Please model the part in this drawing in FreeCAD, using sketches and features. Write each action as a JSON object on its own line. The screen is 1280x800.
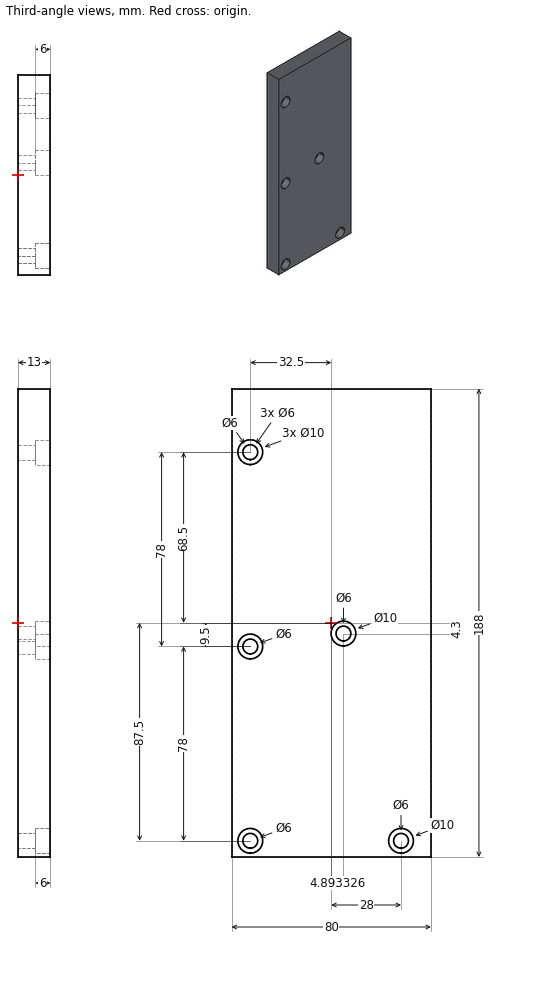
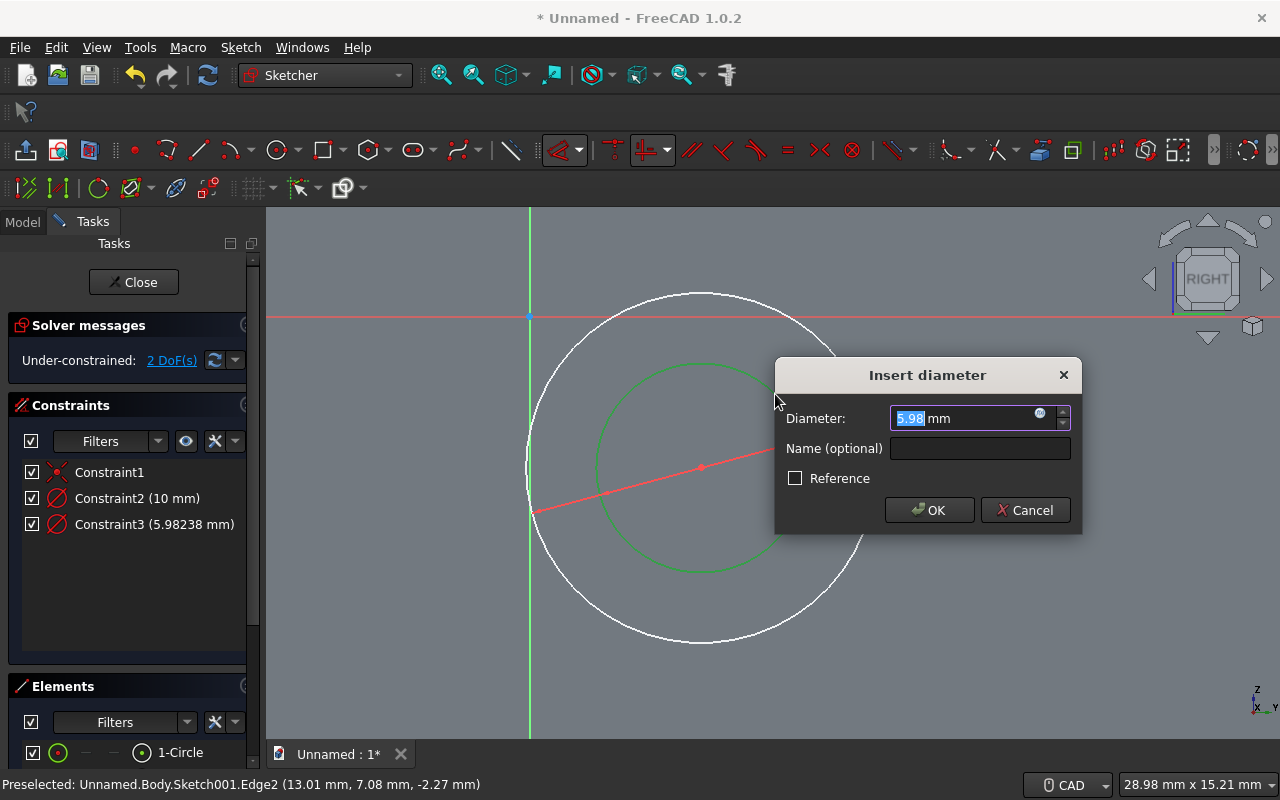
{"action": "type", "text": "6"}
{"action": "key", "text": "Return"}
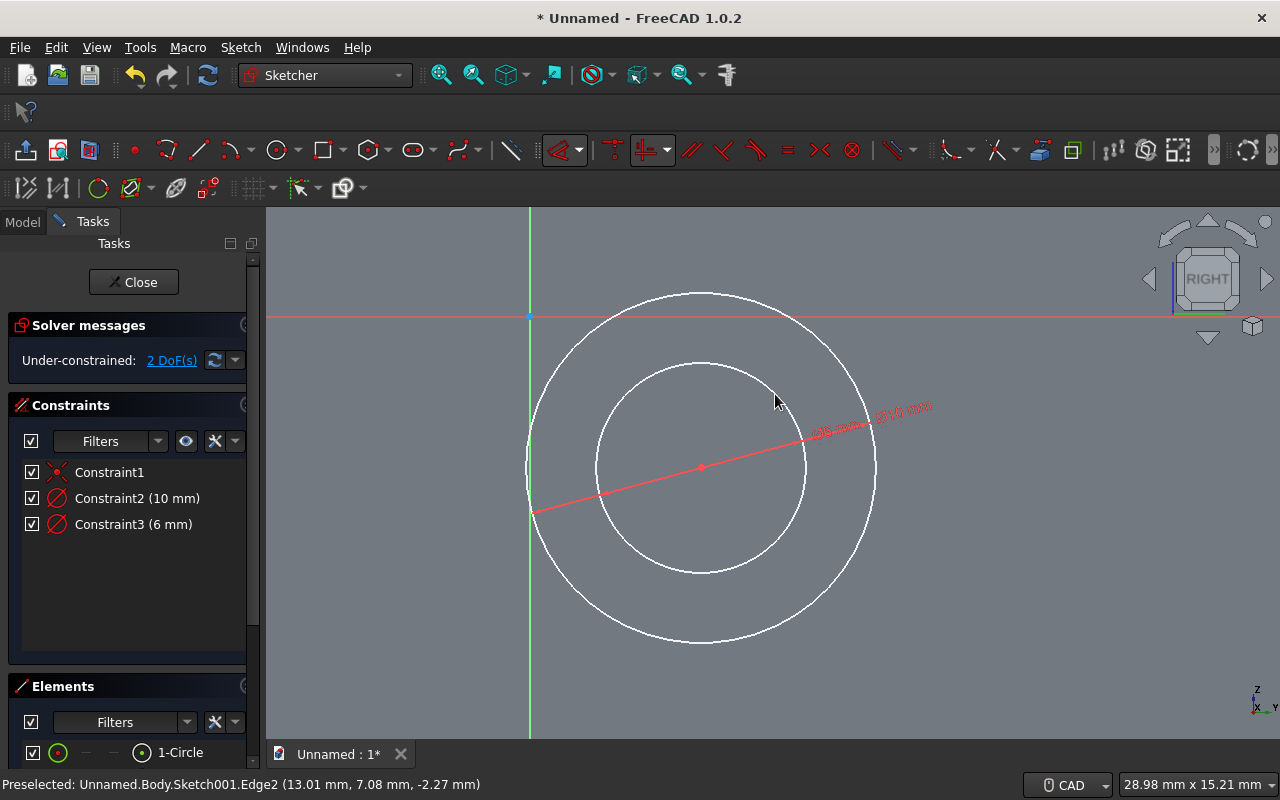
{"action": "left_click", "coordinate": [701, 468]}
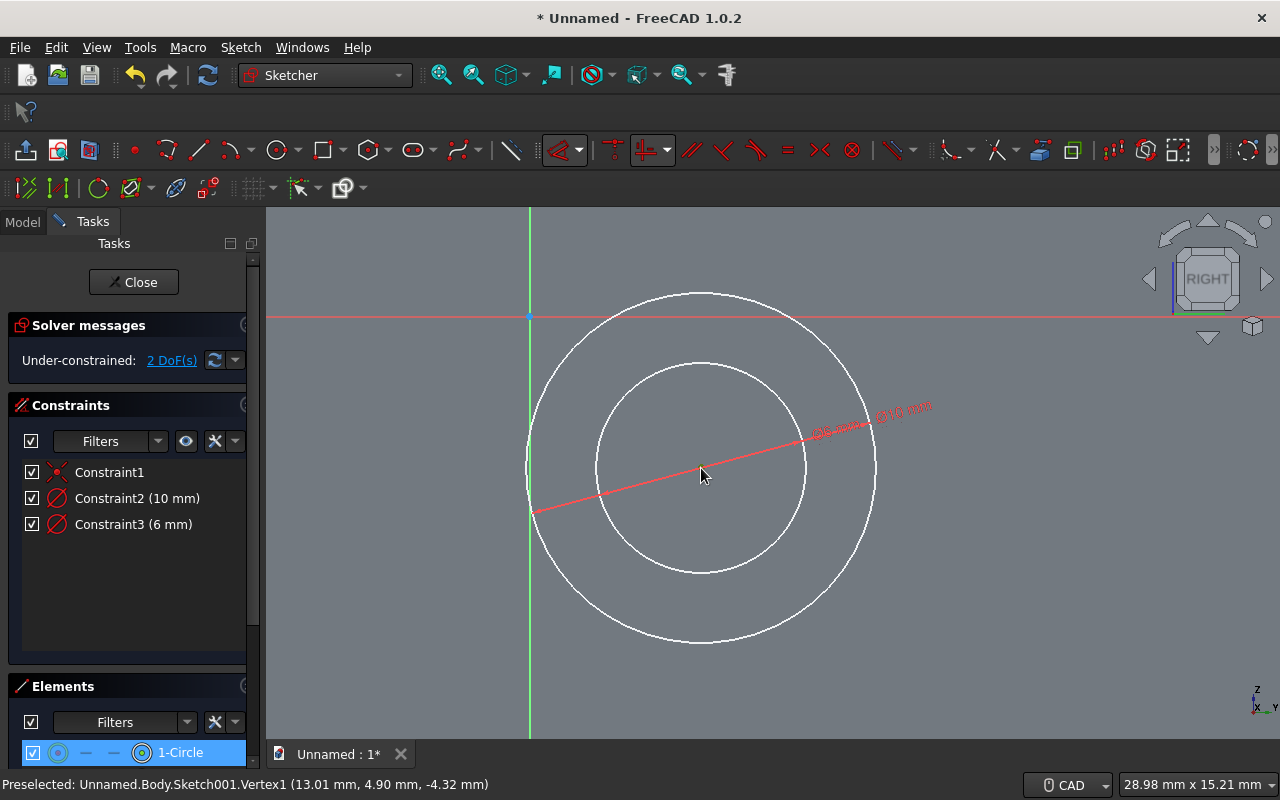
{"action": "key", "text": "i"}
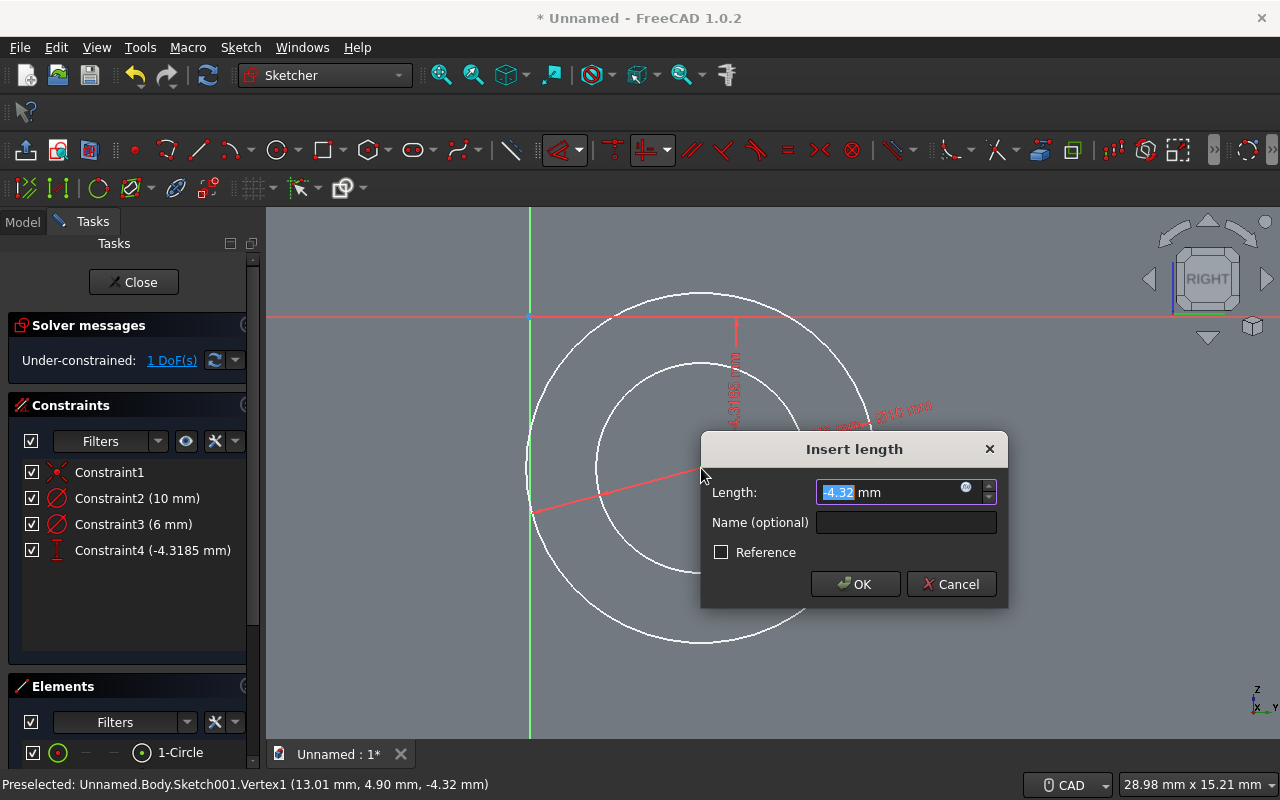
{"action": "type", "text": "-4.3"}
{"action": "key", "text": "Return"}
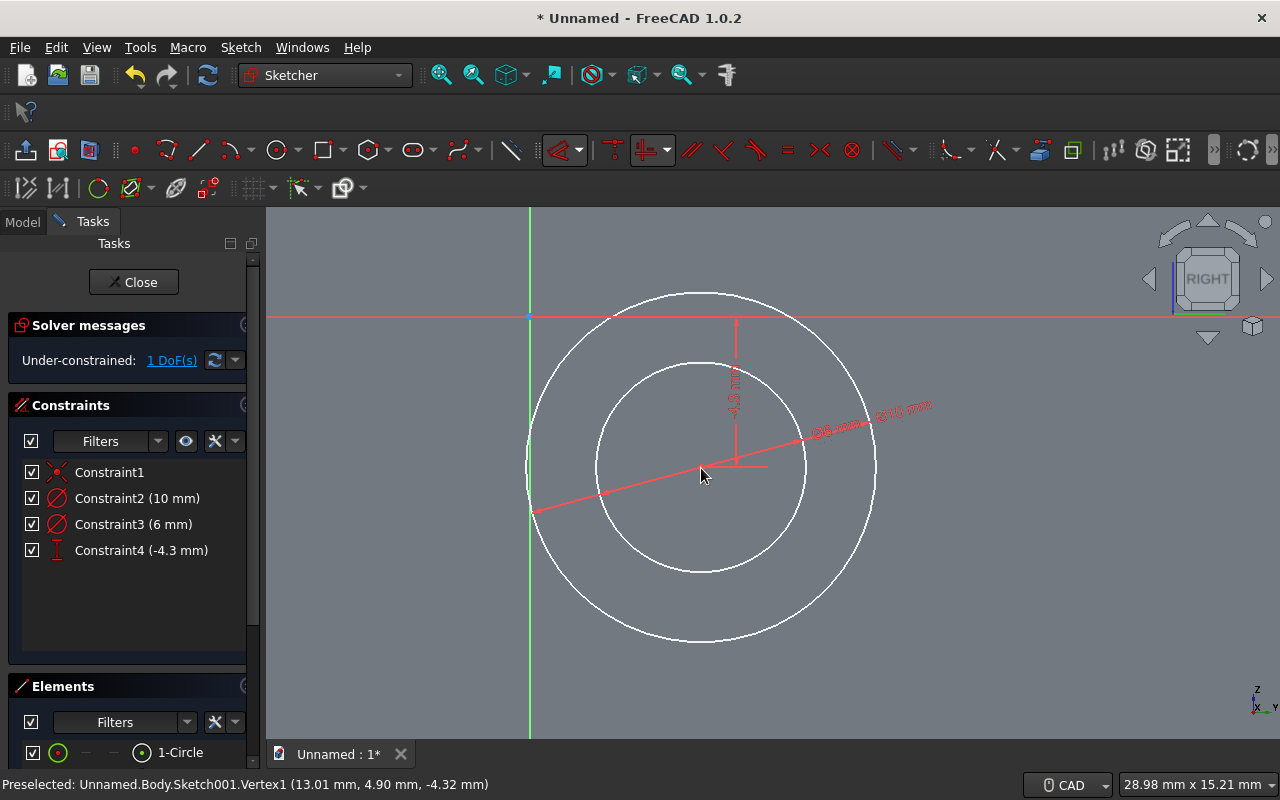
{"action": "left_click", "coordinate": [701, 467]}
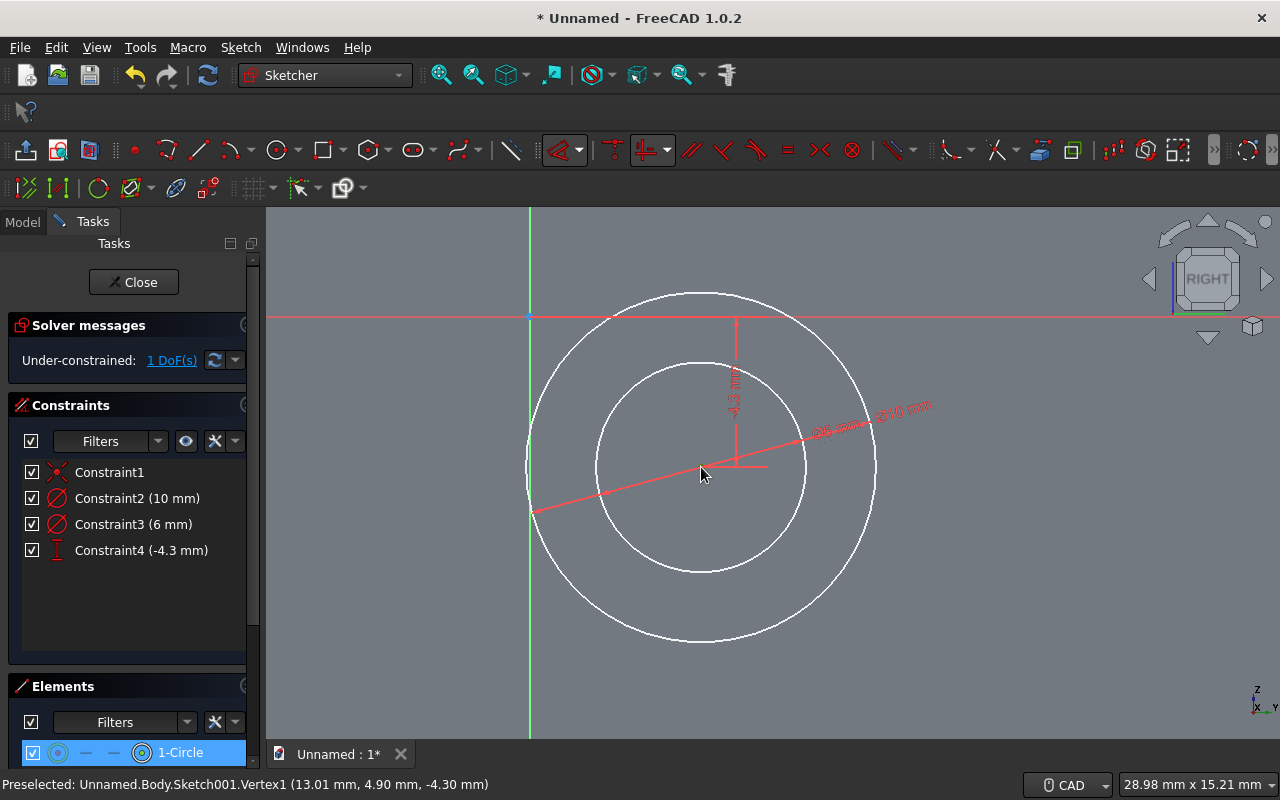
{"action": "left_click", "coordinate": [582, 150]}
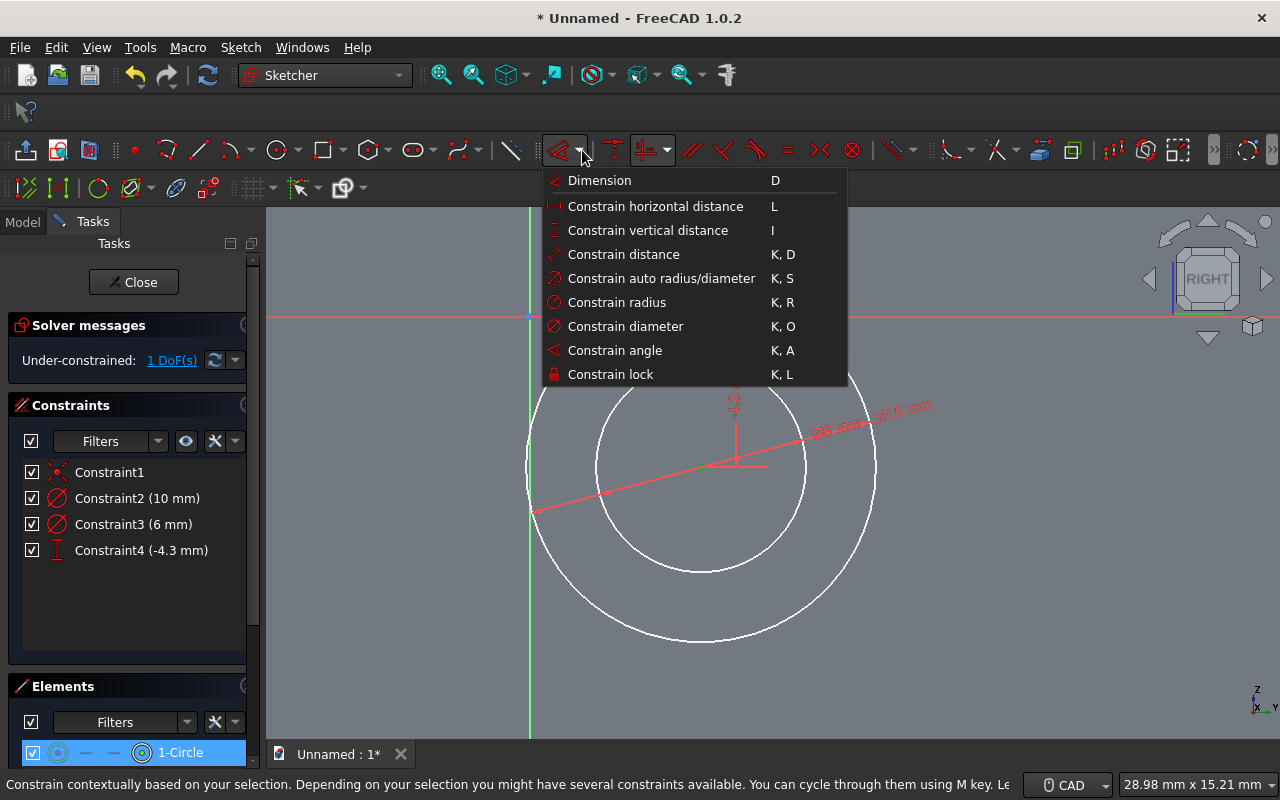
{"action": "left_click", "coordinate": [695, 206]}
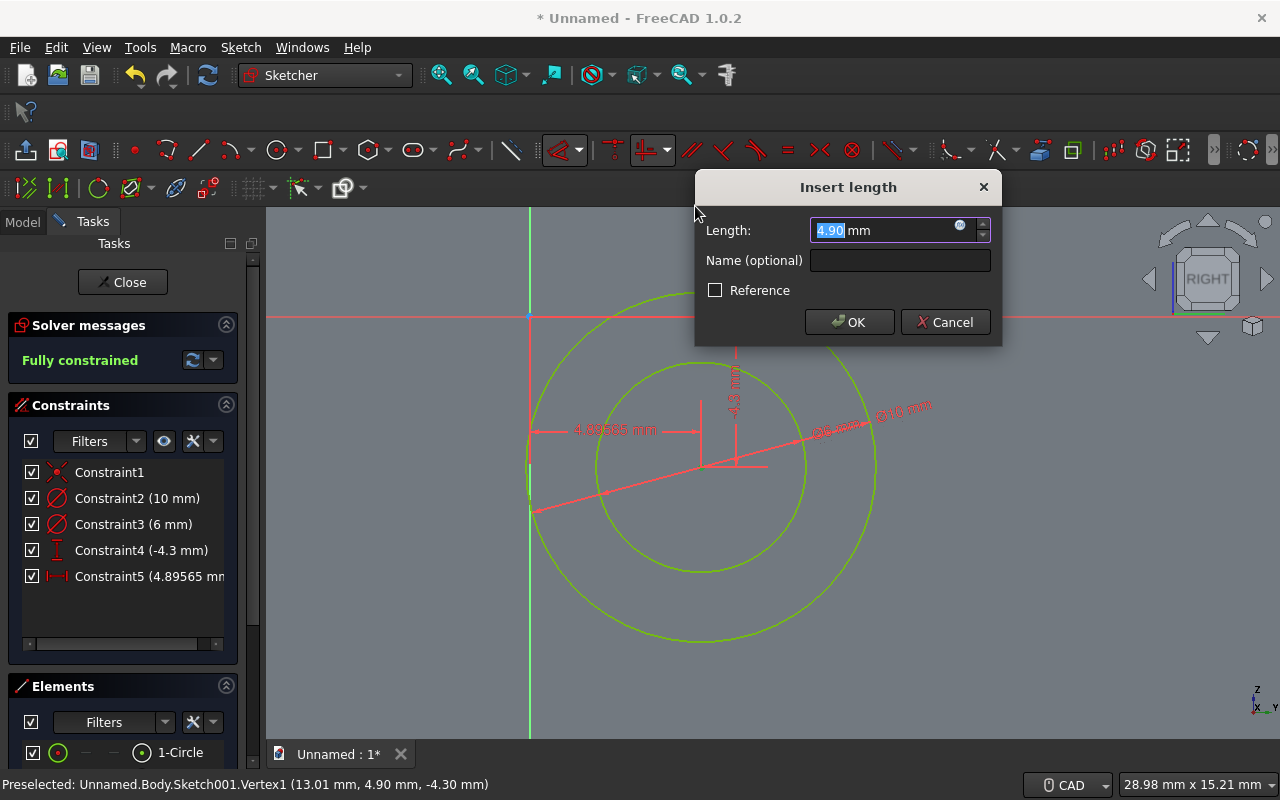
{"action": "type", "text": "4.893326"}
{"action": "key", "text": "Return"}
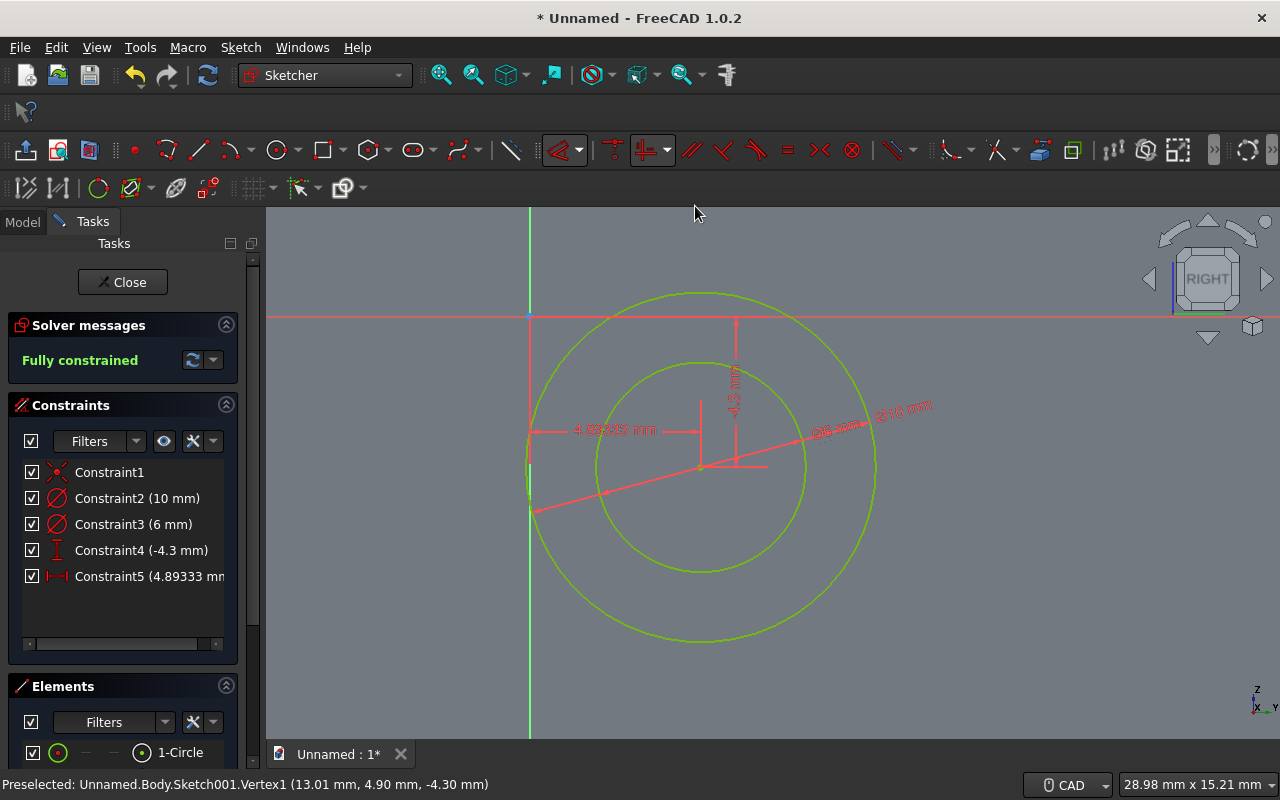
{"action": "left_click", "coordinate": [123, 282]}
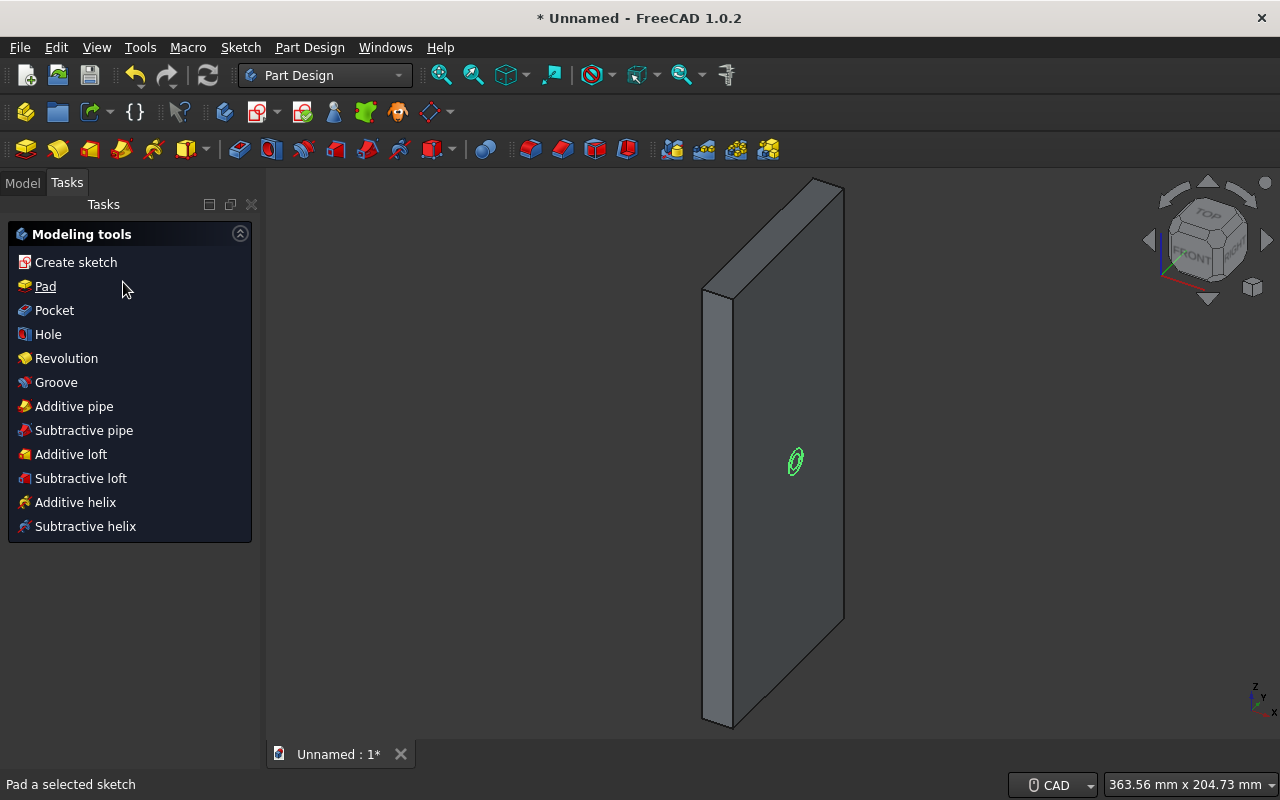
{"action": "left_click", "coordinate": [240, 150]}